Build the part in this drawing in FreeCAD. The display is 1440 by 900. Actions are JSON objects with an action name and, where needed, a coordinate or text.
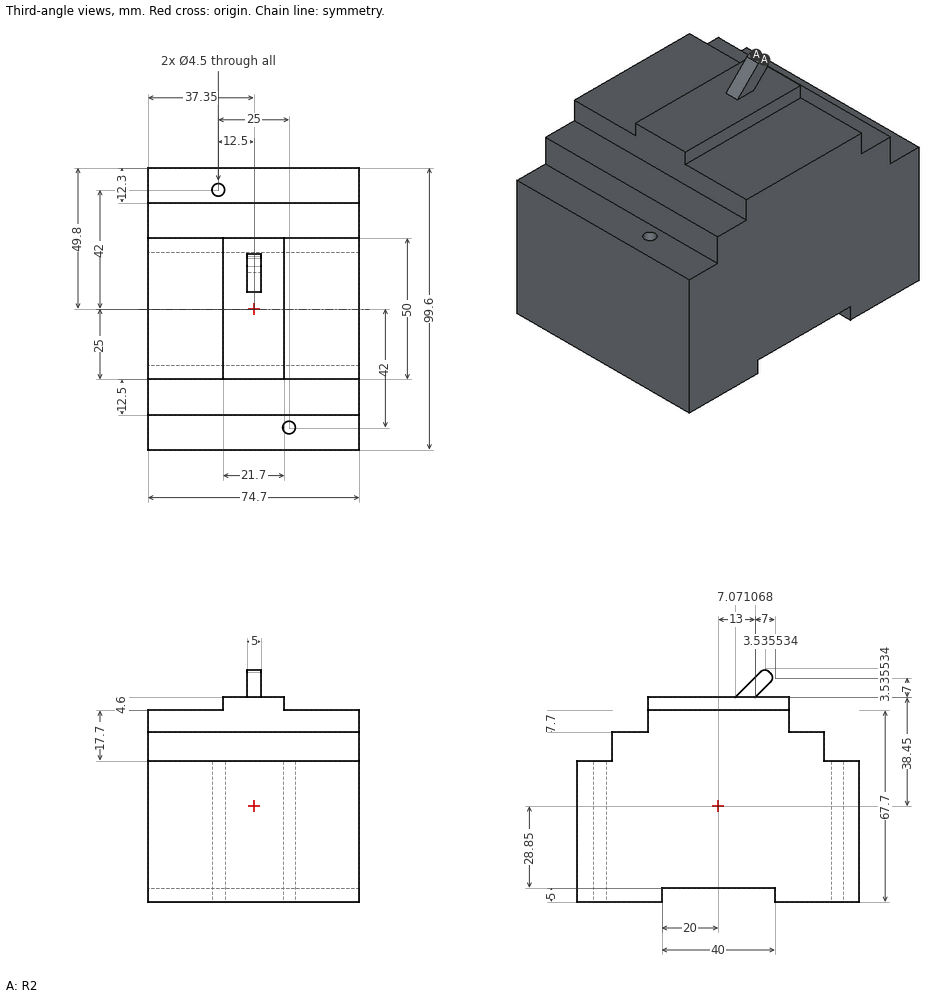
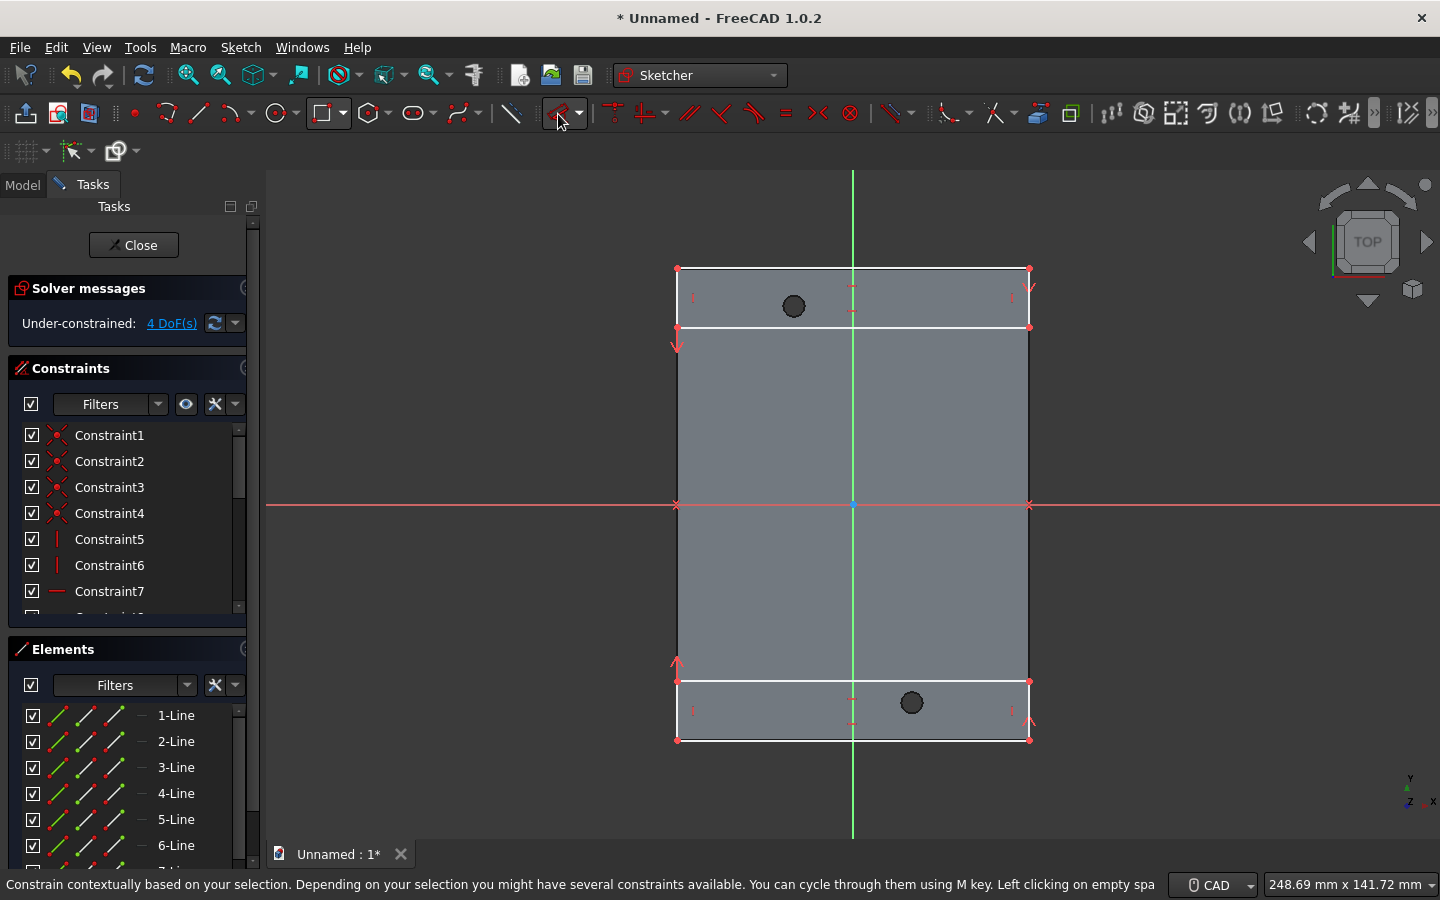
{"action": "left_click", "coordinate": [677, 286]}
{"action": "left_click", "coordinate": [643, 298]}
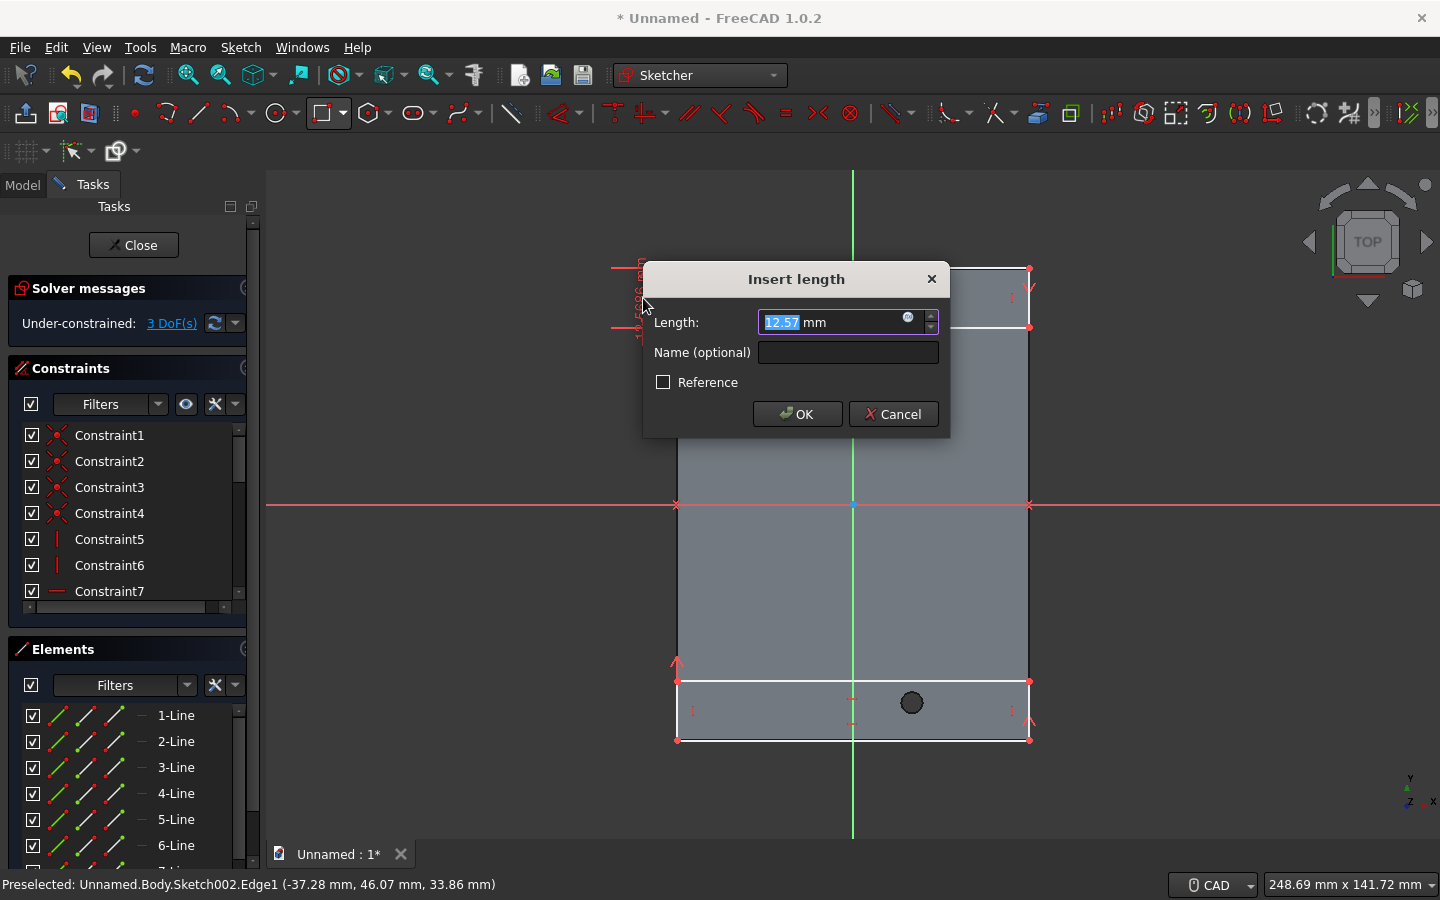
{"action": "type", "text": "12.3"}
{"action": "key", "text": "Return"}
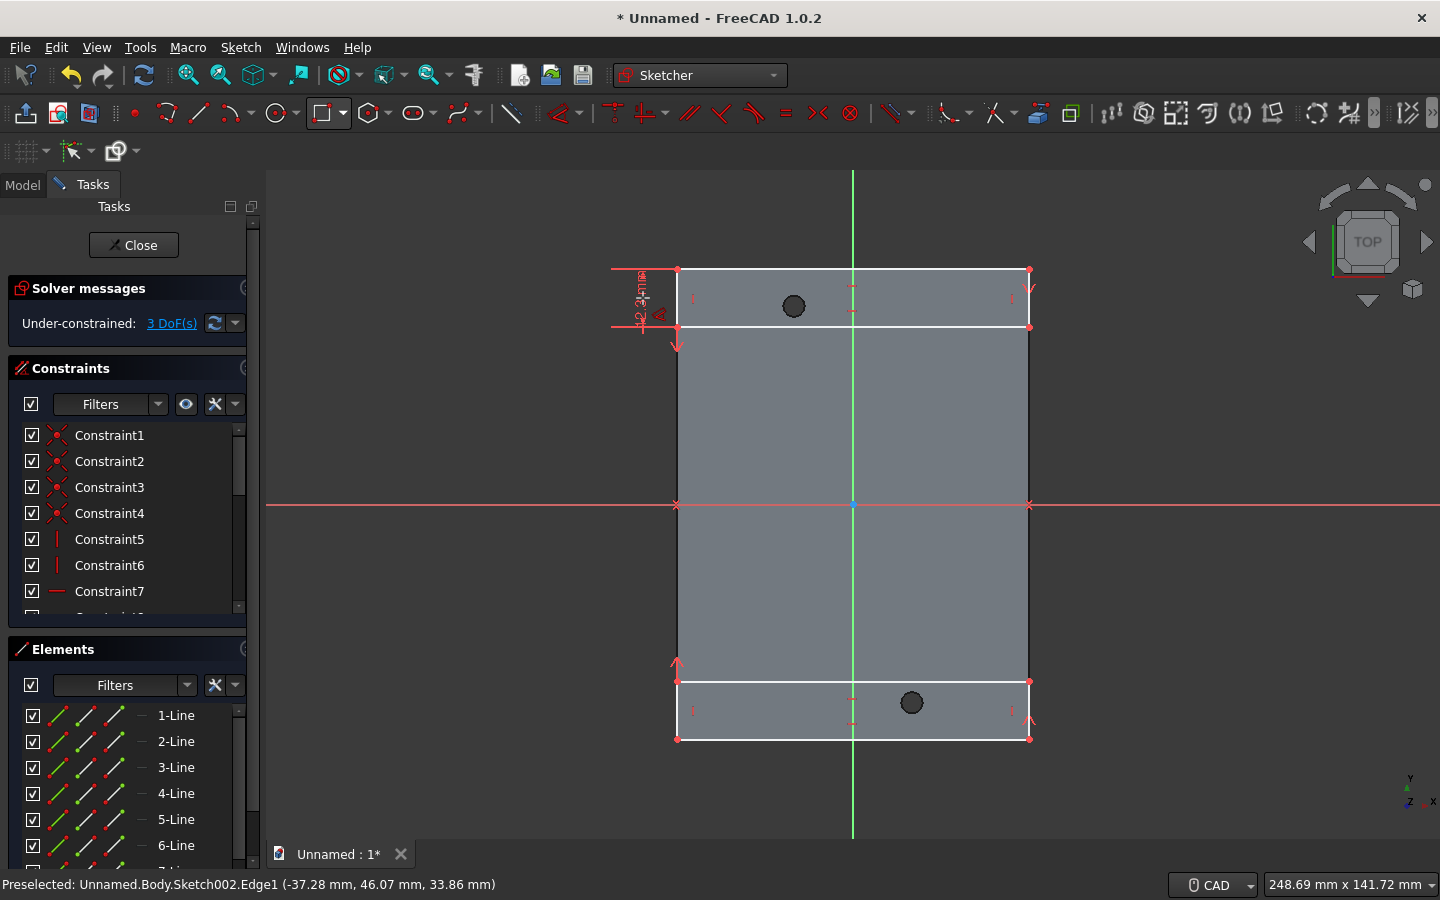
{"action": "left_click", "coordinate": [783, 327]}
{"action": "left_click", "coordinate": [772, 293]}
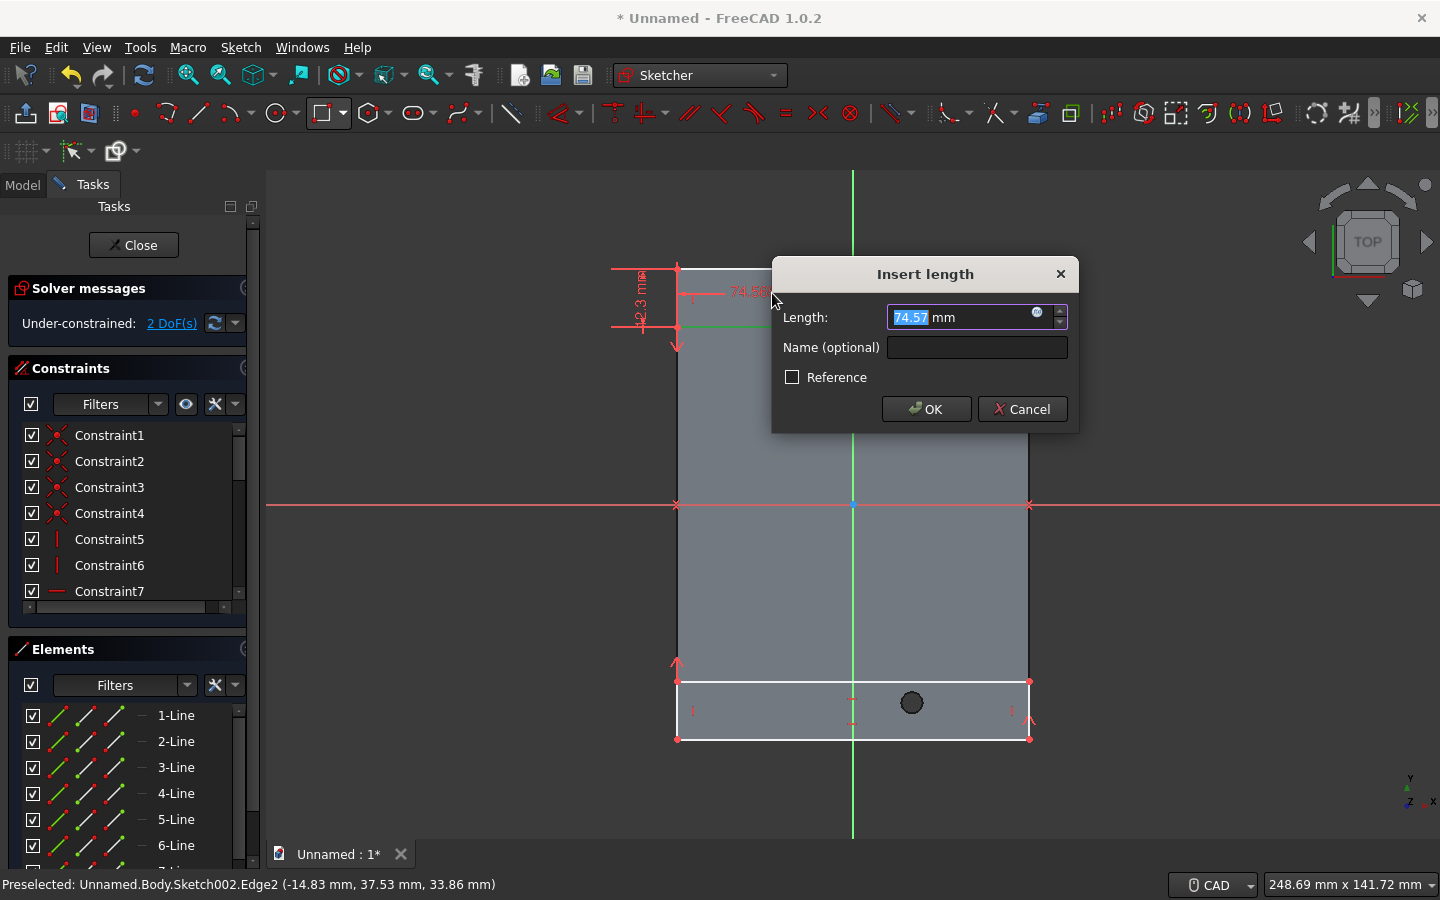
{"action": "type", "text": "74.7"}
{"action": "key", "text": "Return"}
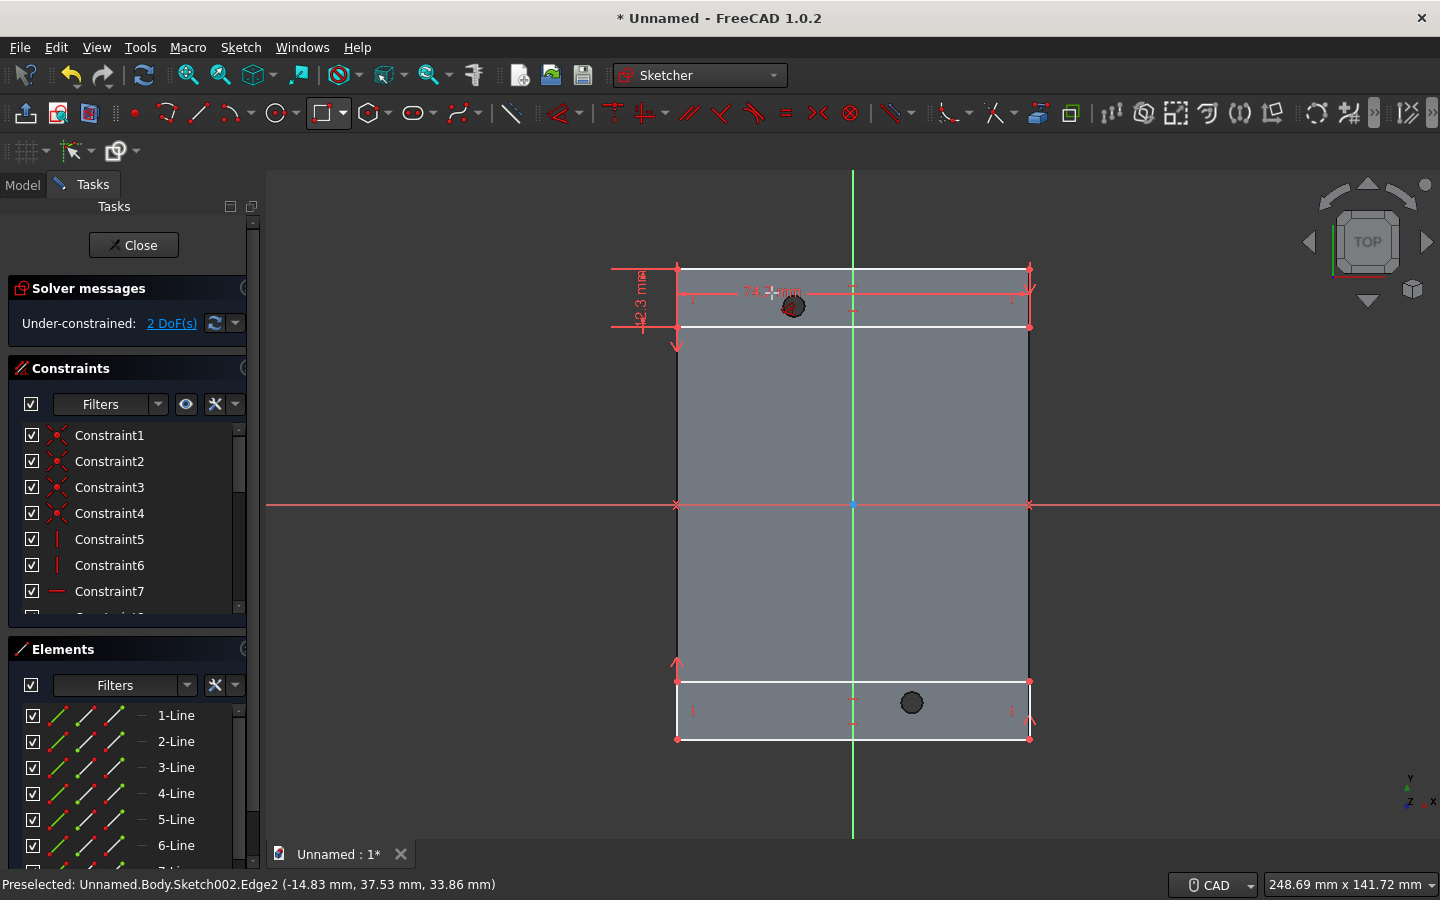
{"action": "left_click", "coordinate": [677, 269]}
{"action": "left_click", "coordinate": [643, 387]}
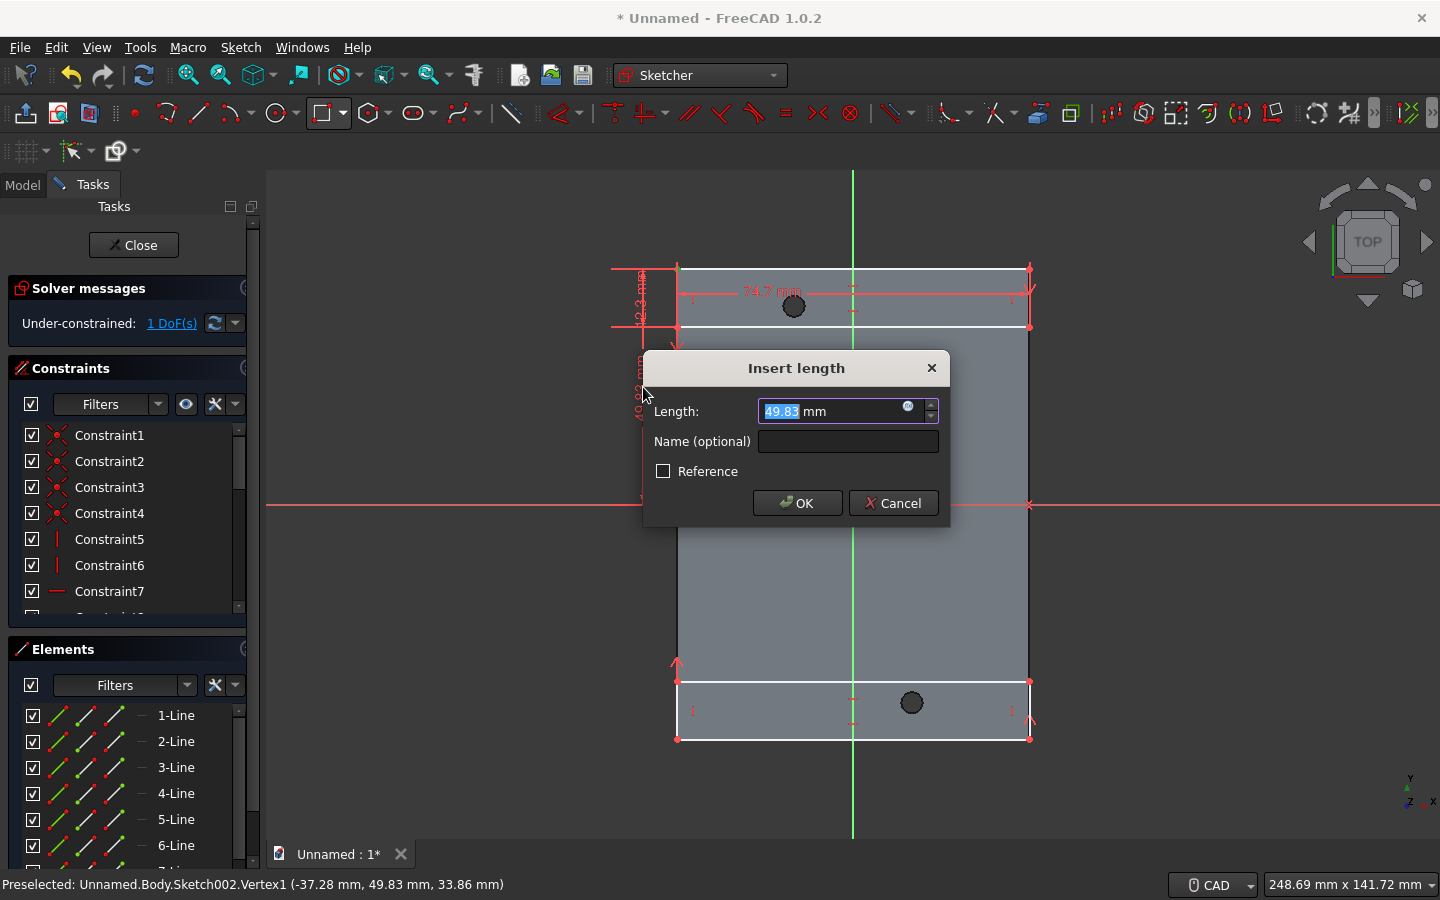
{"action": "type", "text": "49.8"}
{"action": "key", "text": "Return"}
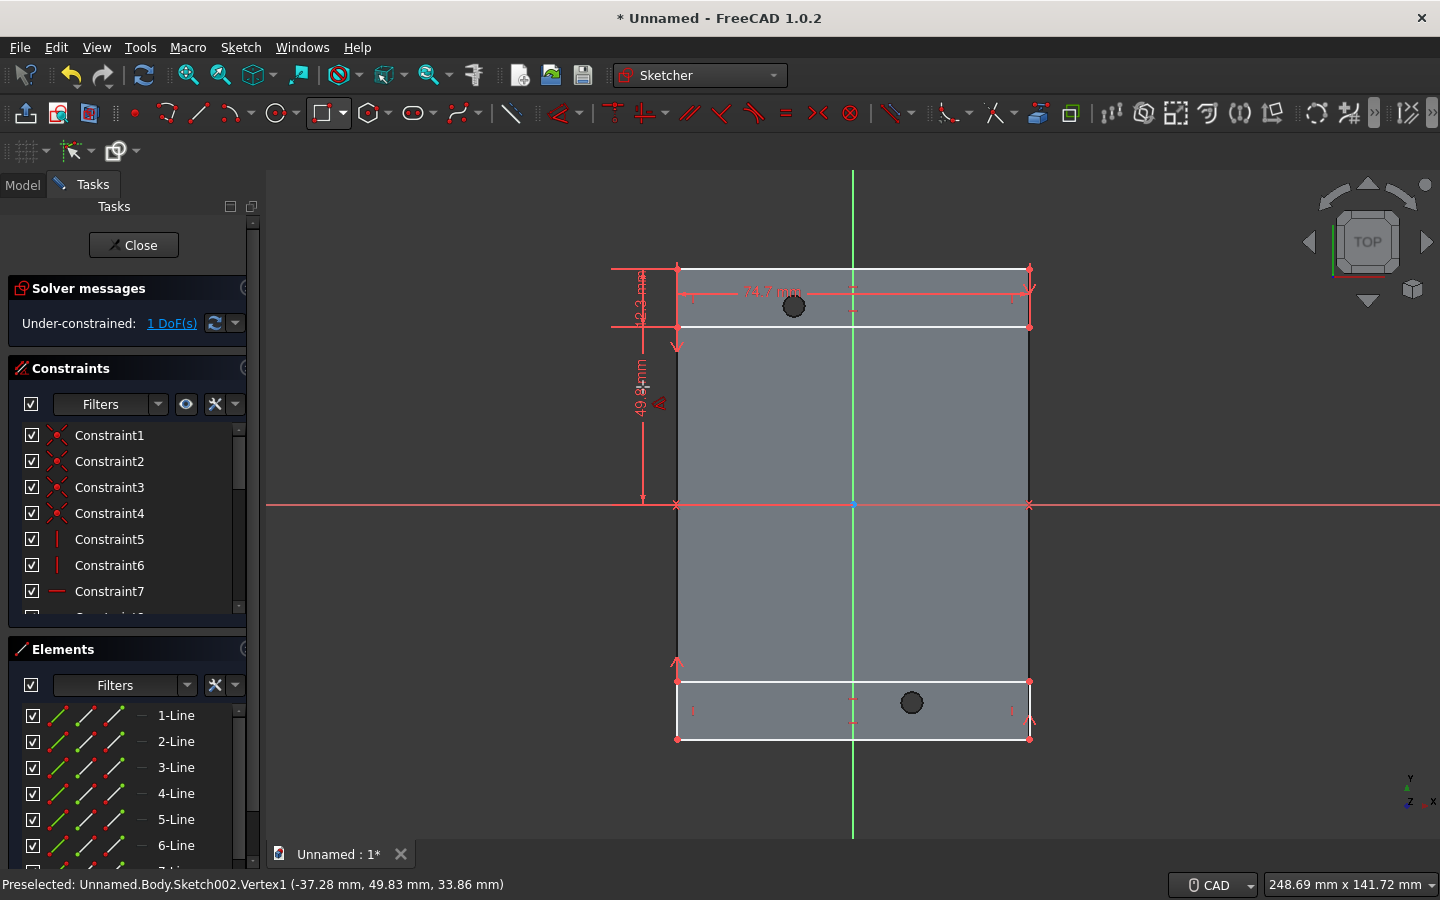
{"action": "left_click", "coordinate": [677, 269]}
{"action": "left_click", "coordinate": [765, 235]}